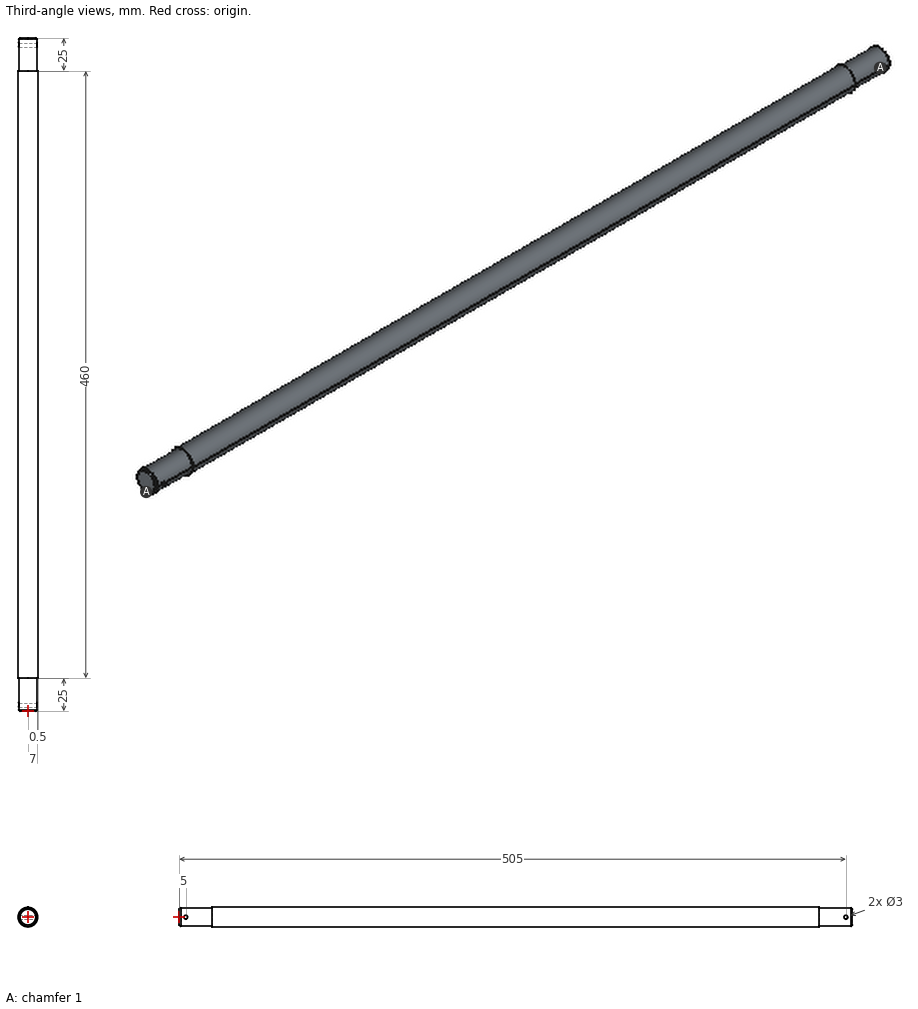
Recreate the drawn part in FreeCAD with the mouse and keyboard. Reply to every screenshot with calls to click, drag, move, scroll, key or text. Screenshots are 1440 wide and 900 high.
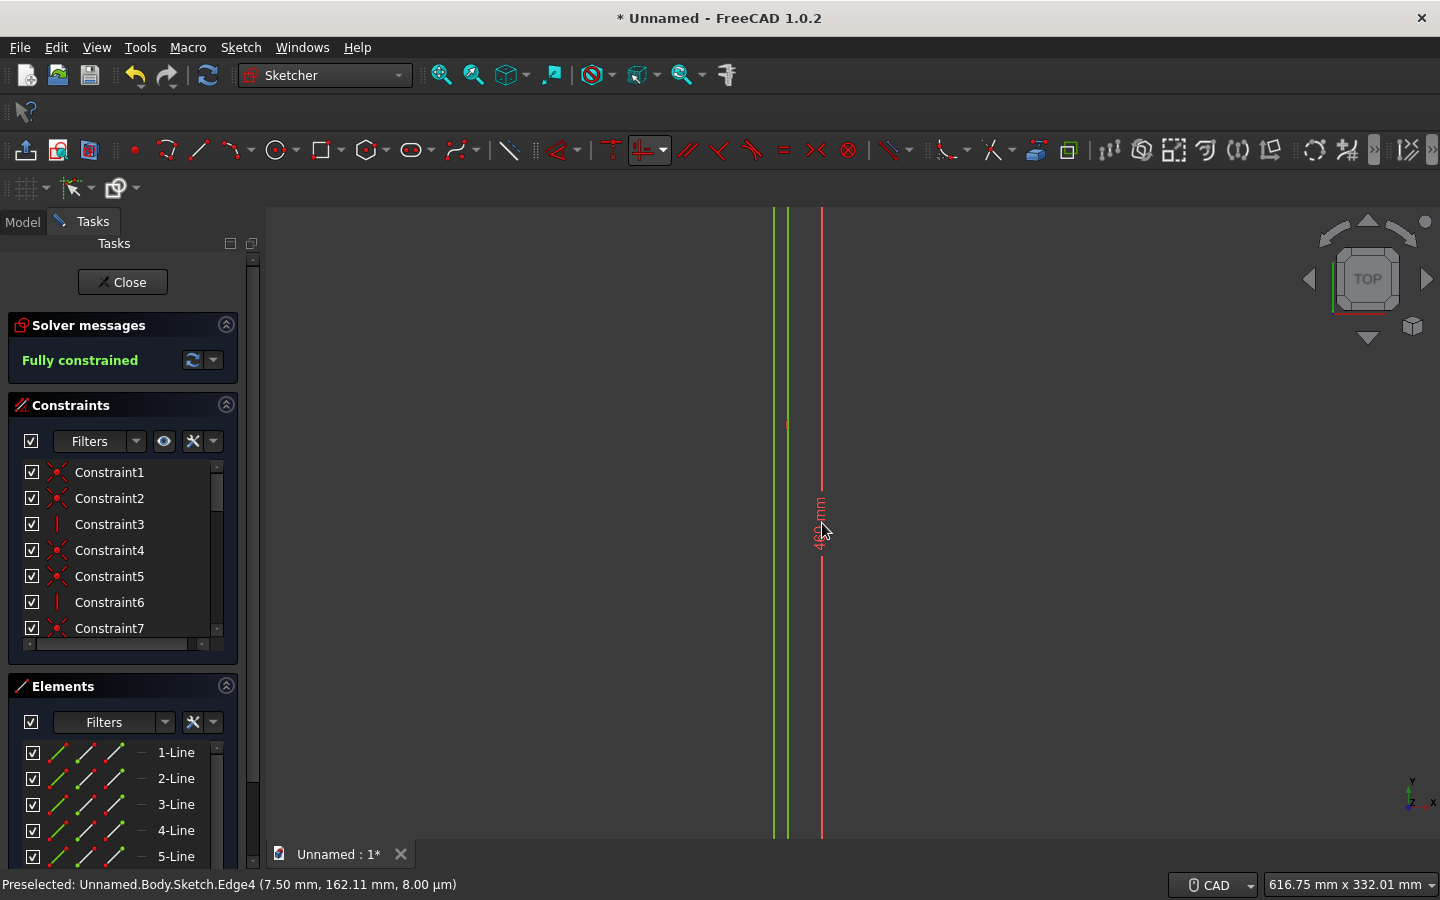
click(123, 282)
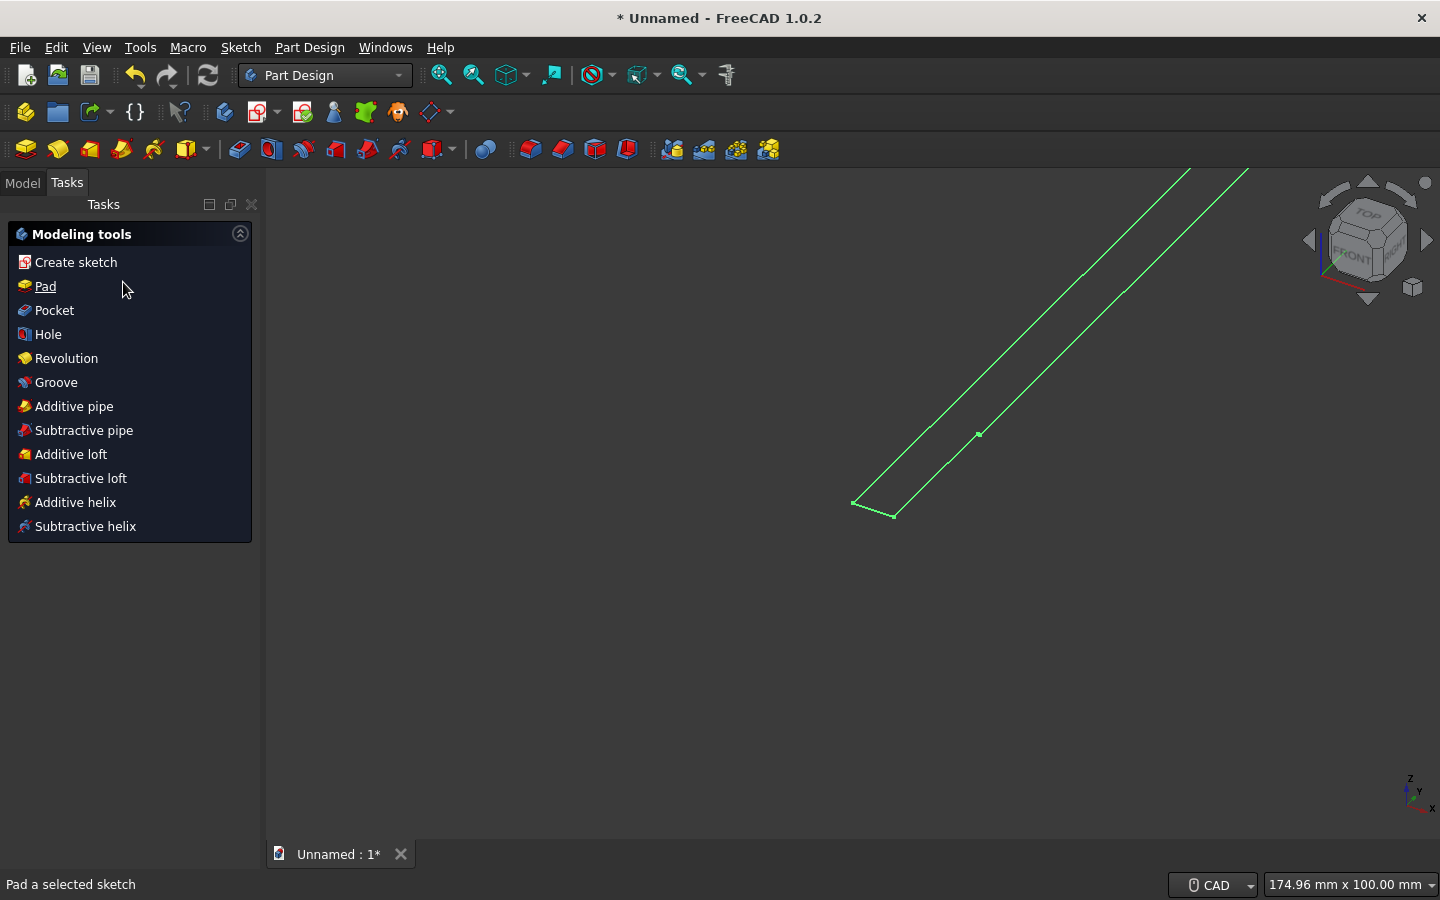
click(58, 150)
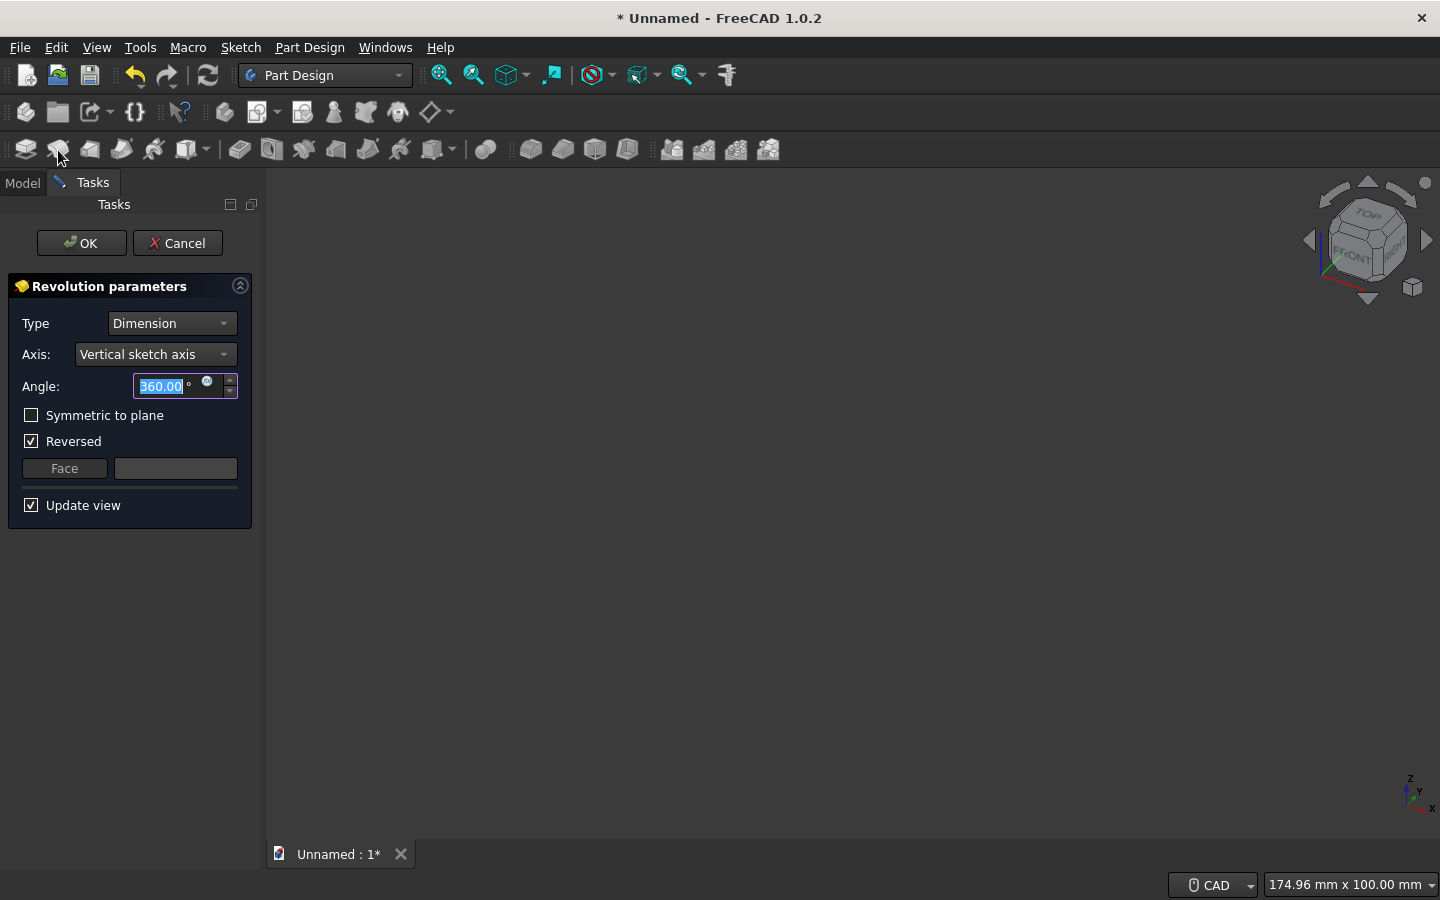
click(82, 243)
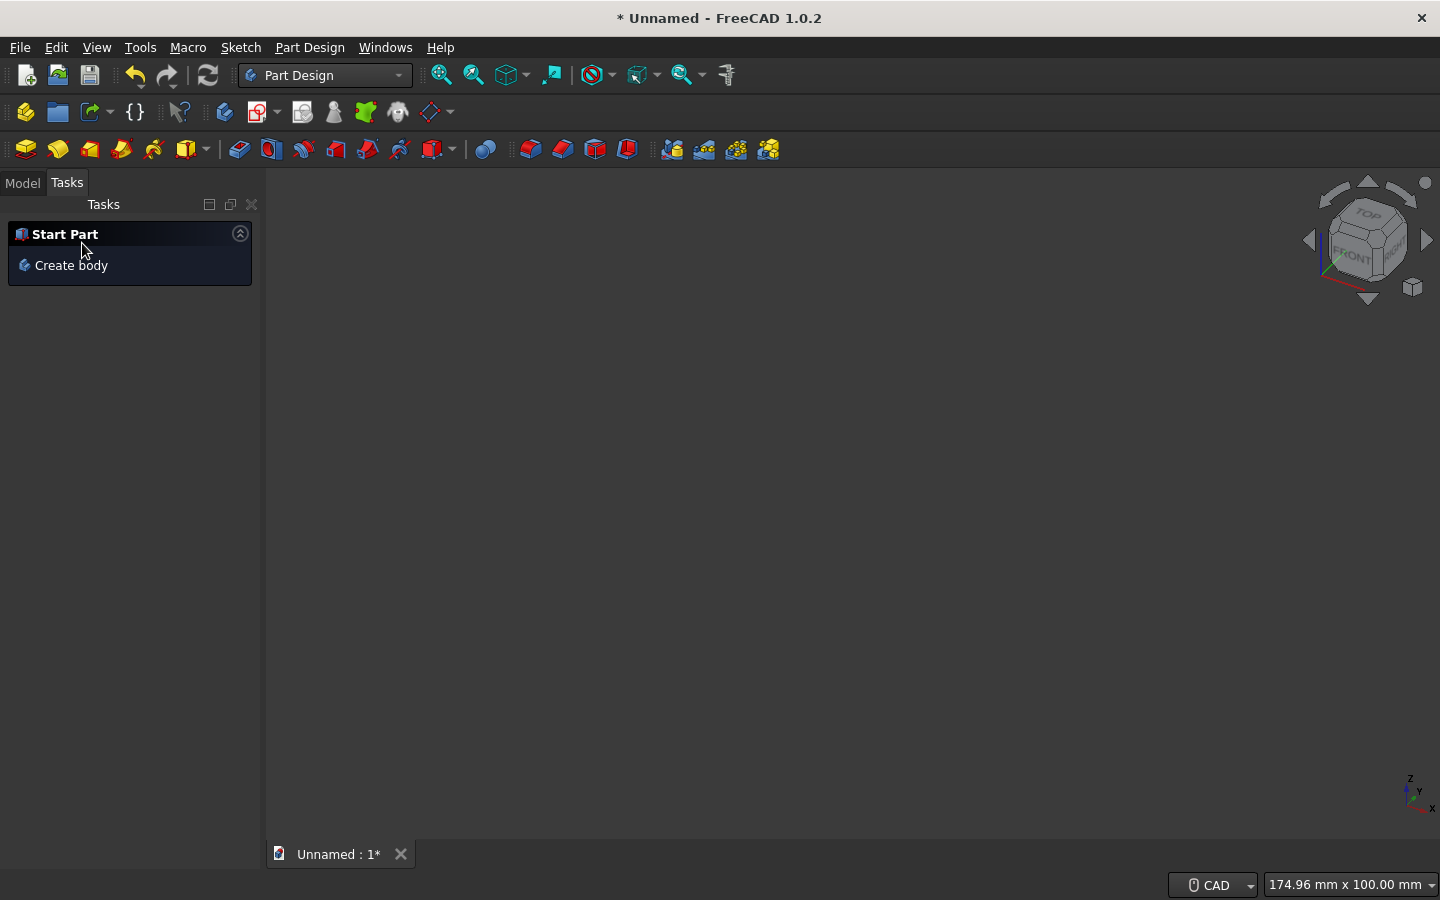
click(442, 76)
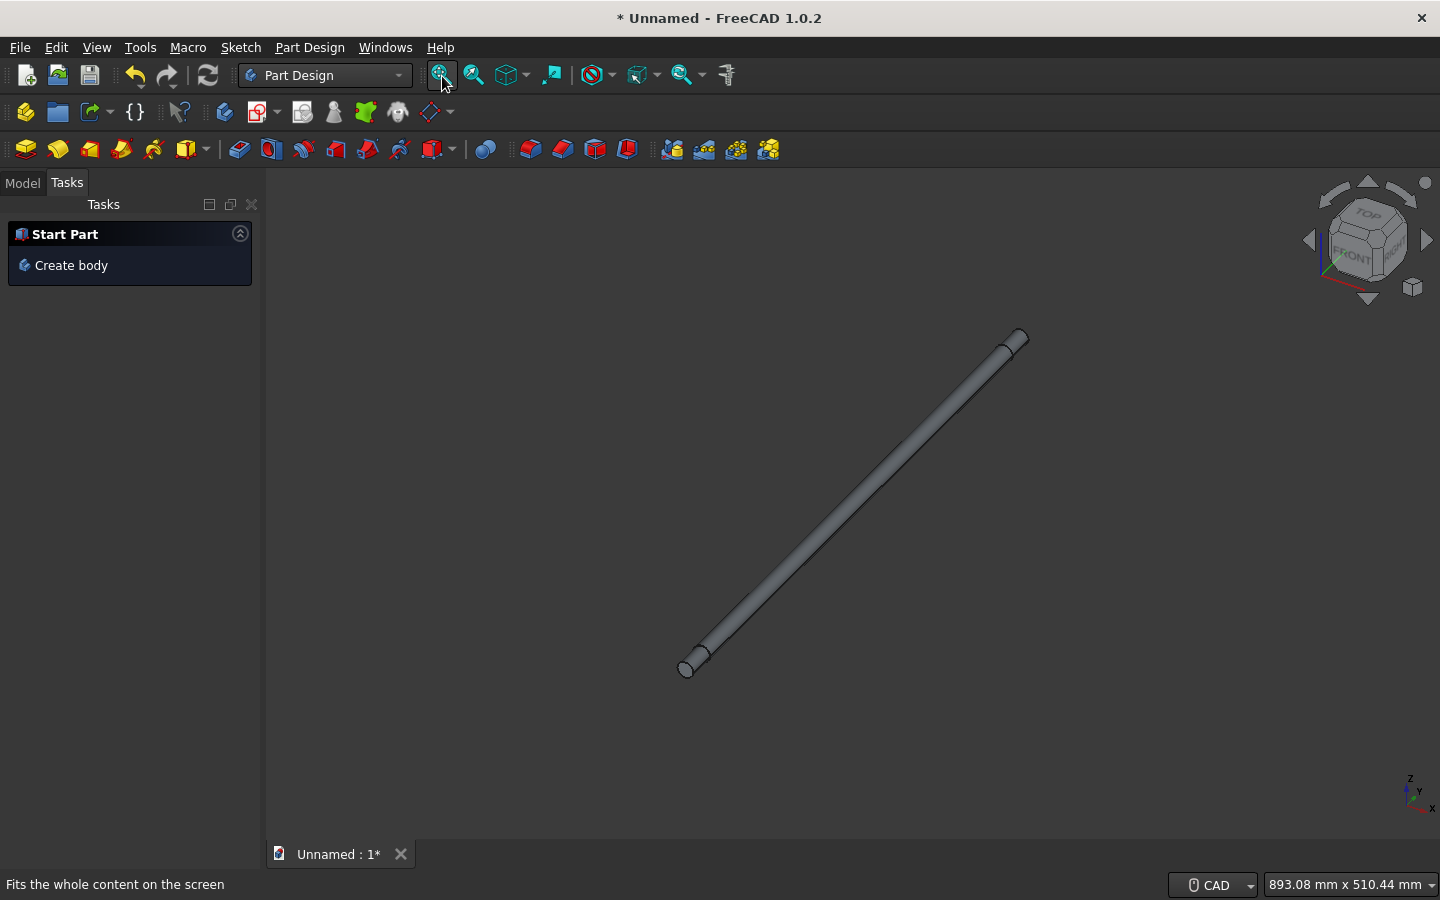
click(1018, 328)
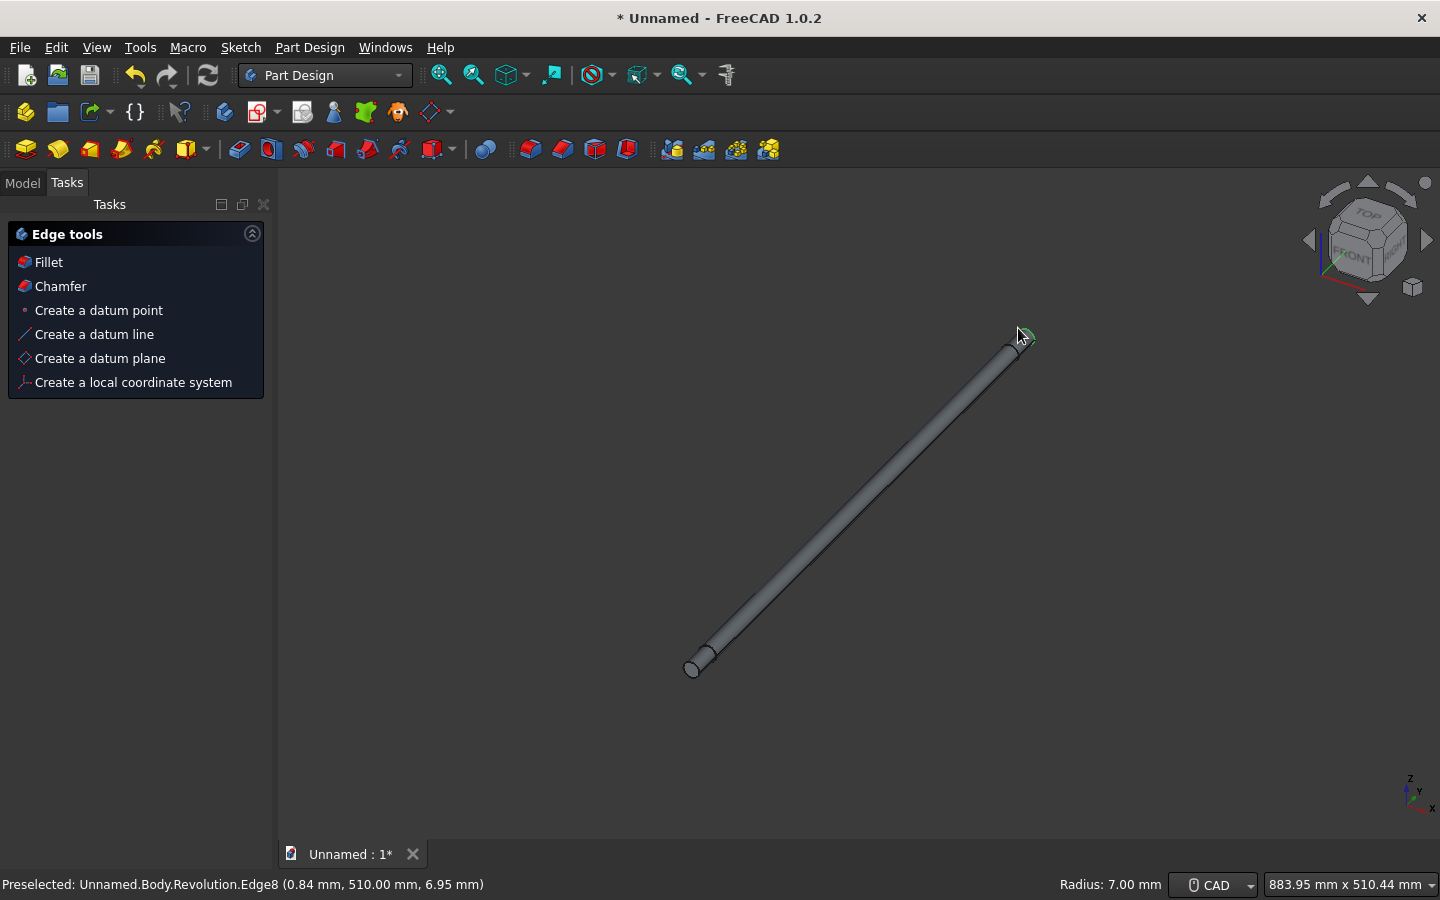
click(683, 666, ctrl)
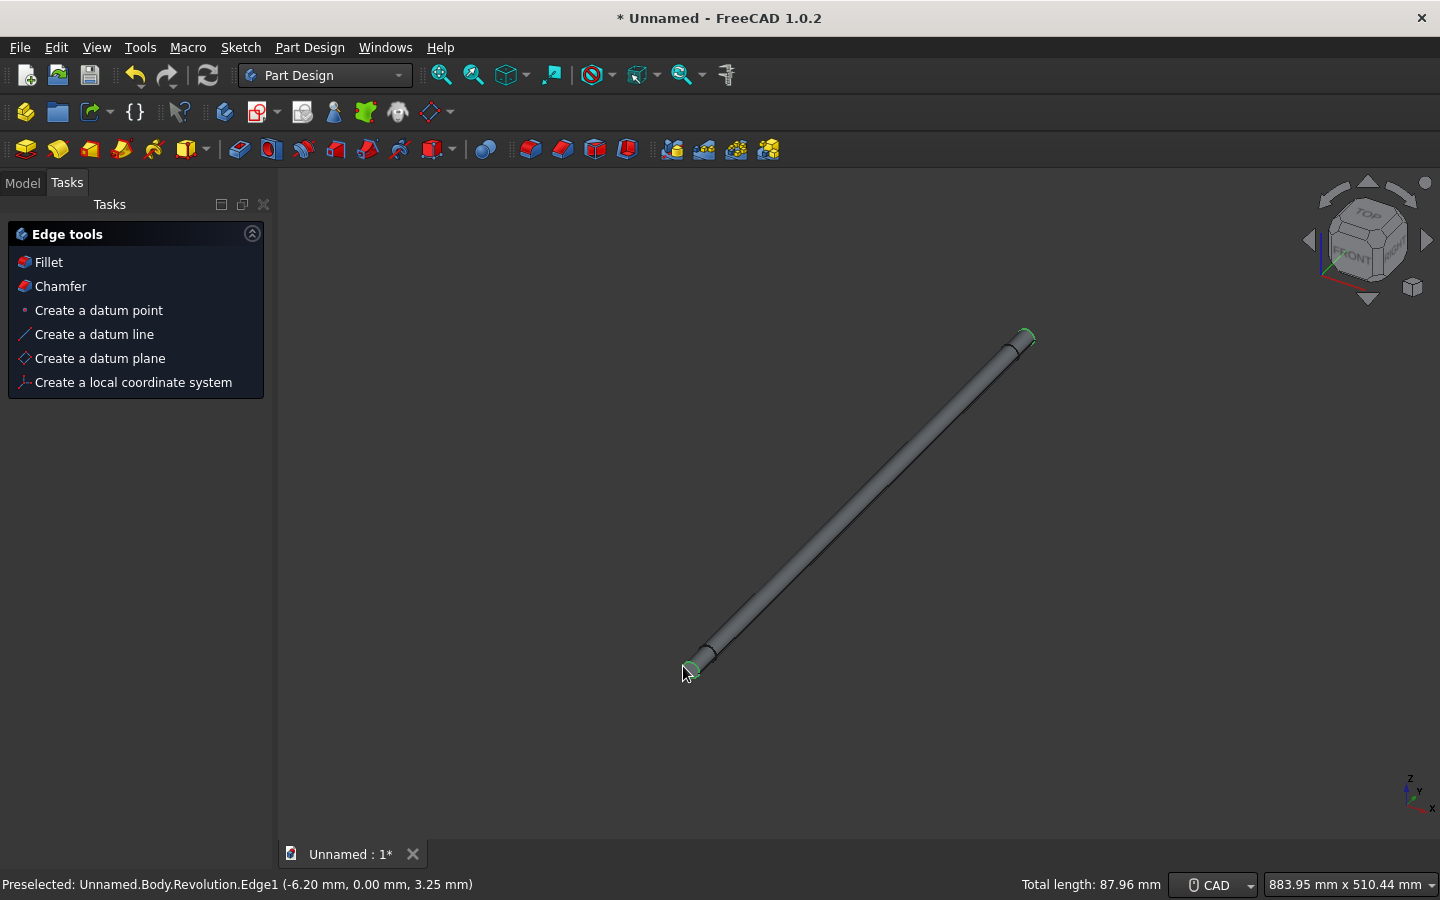
click(564, 150)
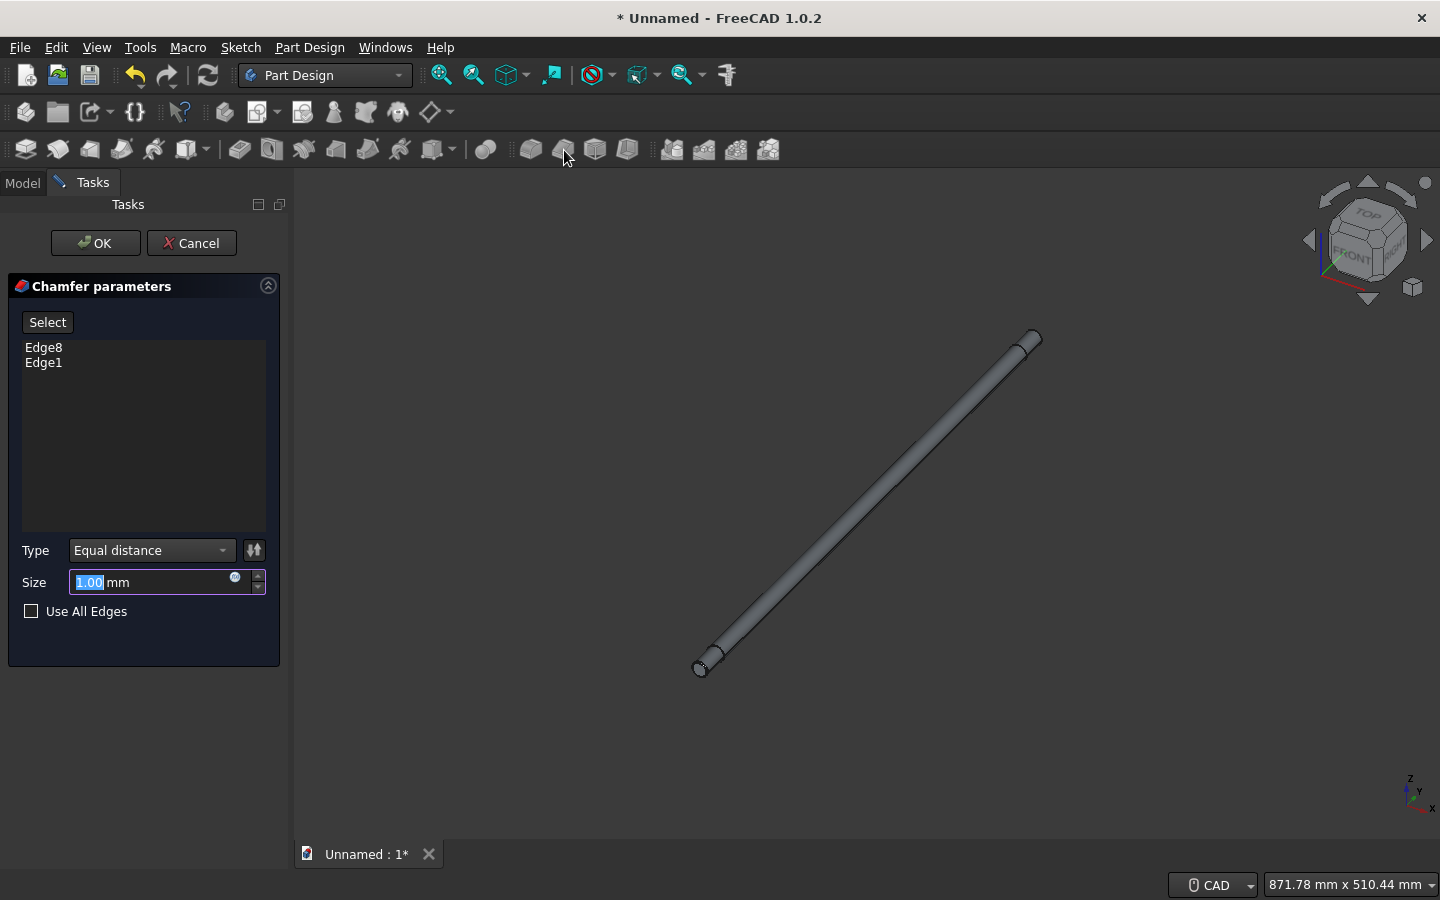
text(1)
key(Tab)